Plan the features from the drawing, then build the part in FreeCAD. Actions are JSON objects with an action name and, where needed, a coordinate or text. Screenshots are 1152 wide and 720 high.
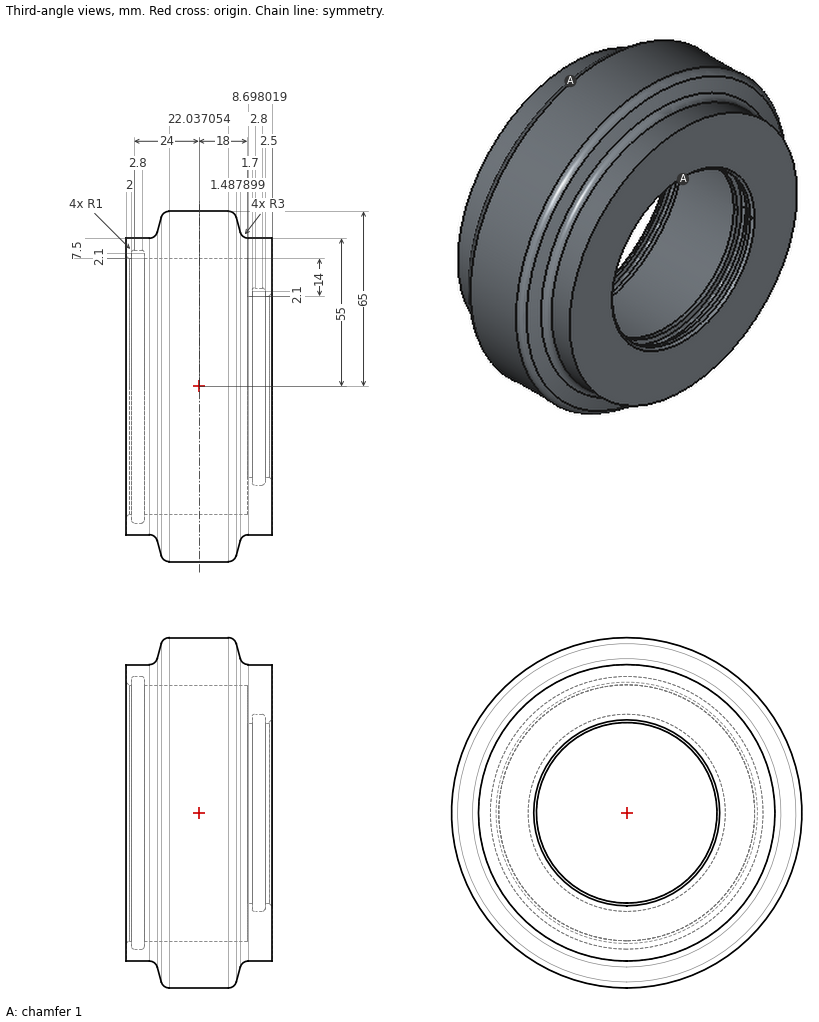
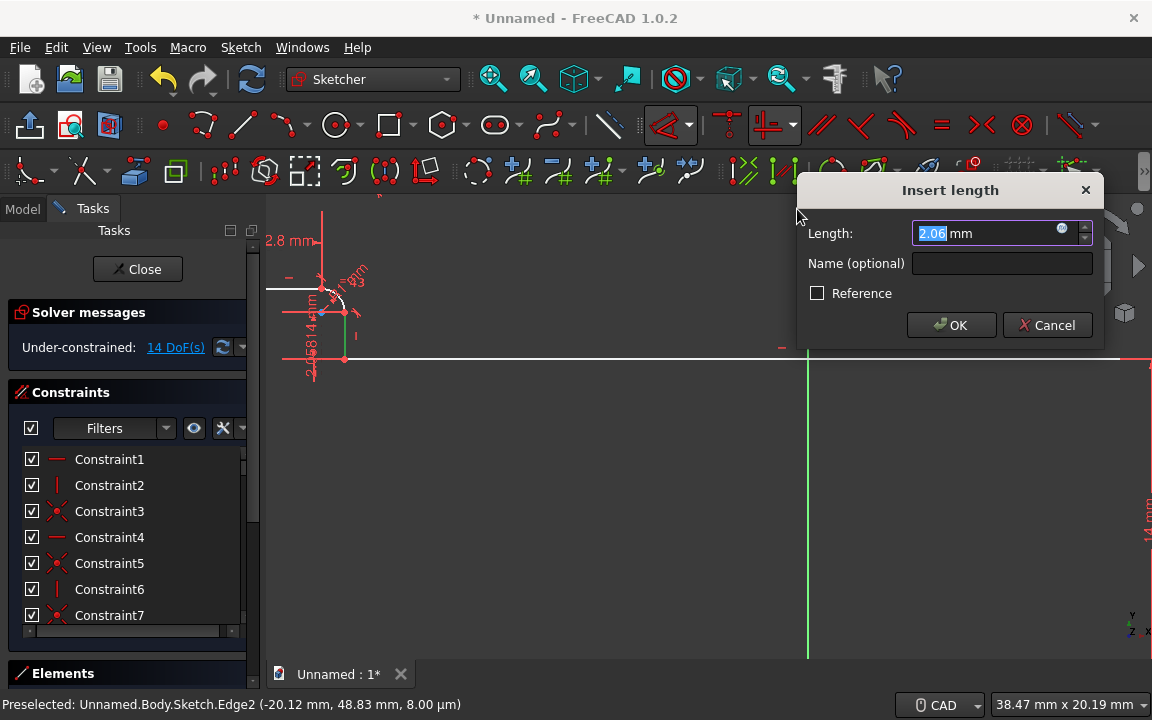
{"action": "type", "text": "2.1"}
{"action": "key", "text": "Return"}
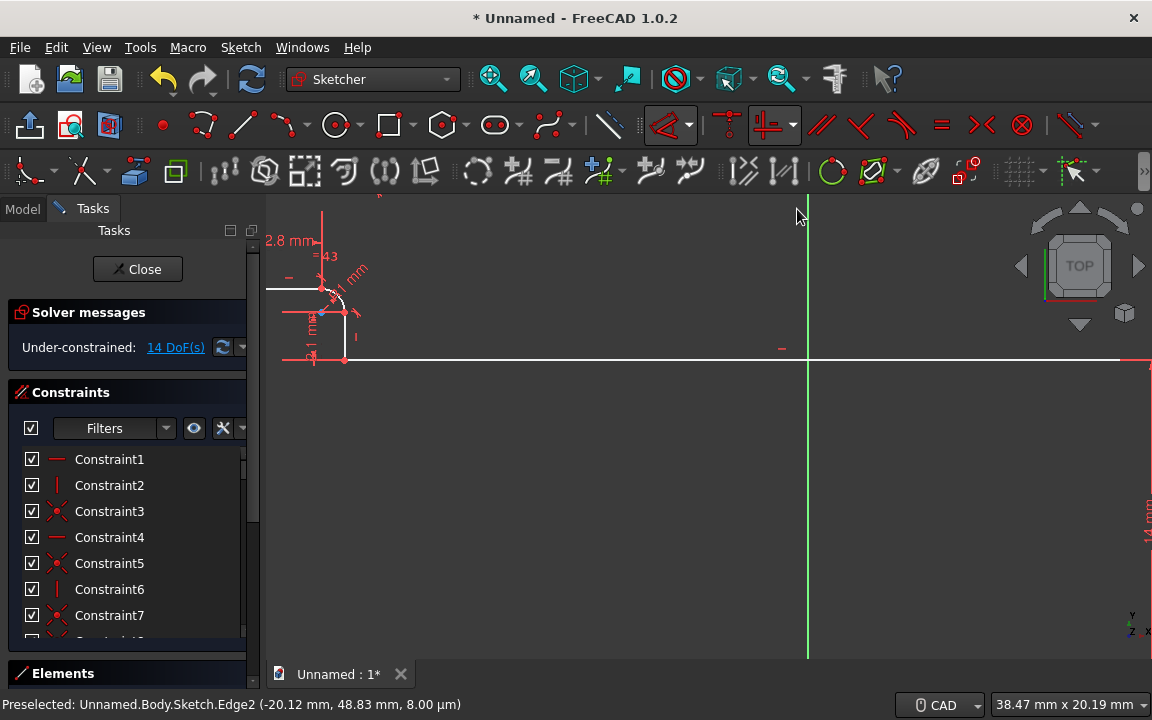
{"action": "scroll", "coordinate": [598, 357], "scroll_direction": "down", "scroll_amount": 8}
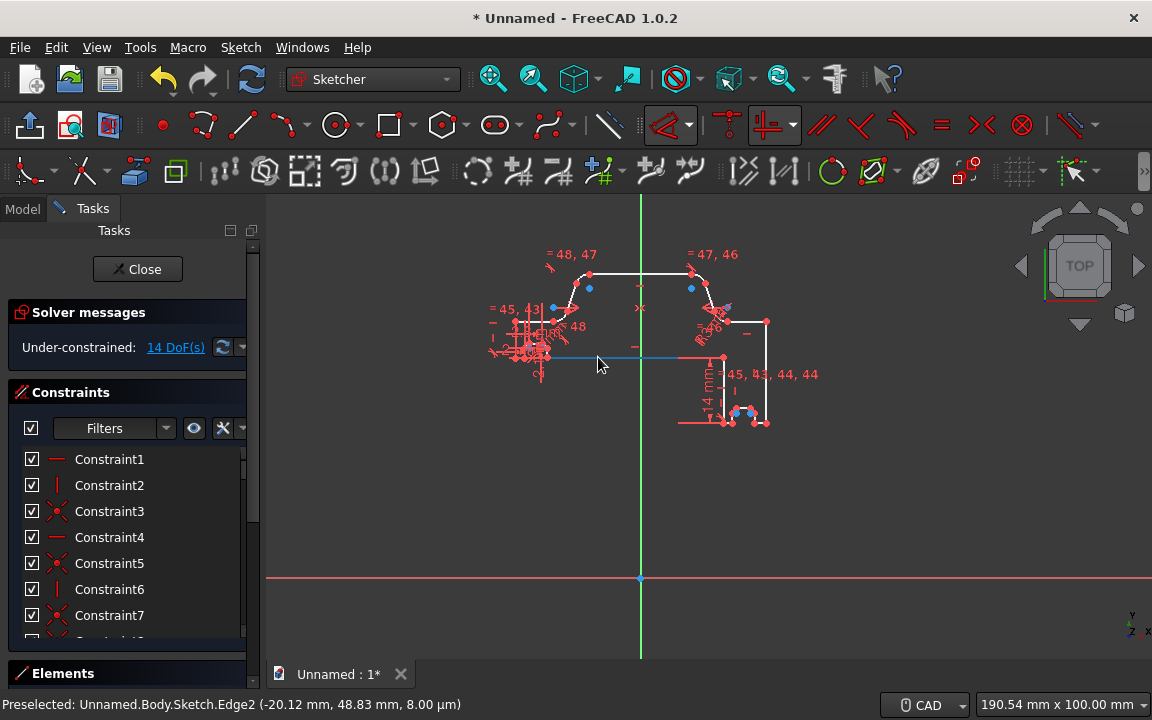
{"action": "scroll", "coordinate": [726, 423], "scroll_direction": "up", "scroll_amount": 9}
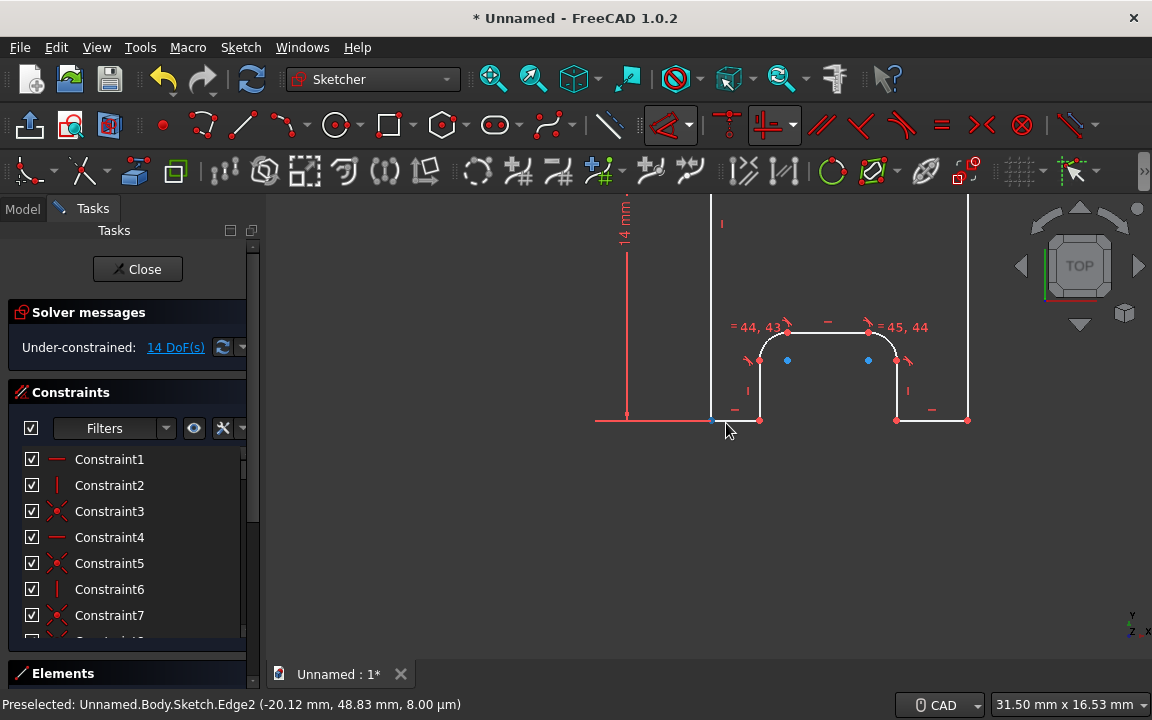
{"action": "left_click", "coordinate": [726, 421]}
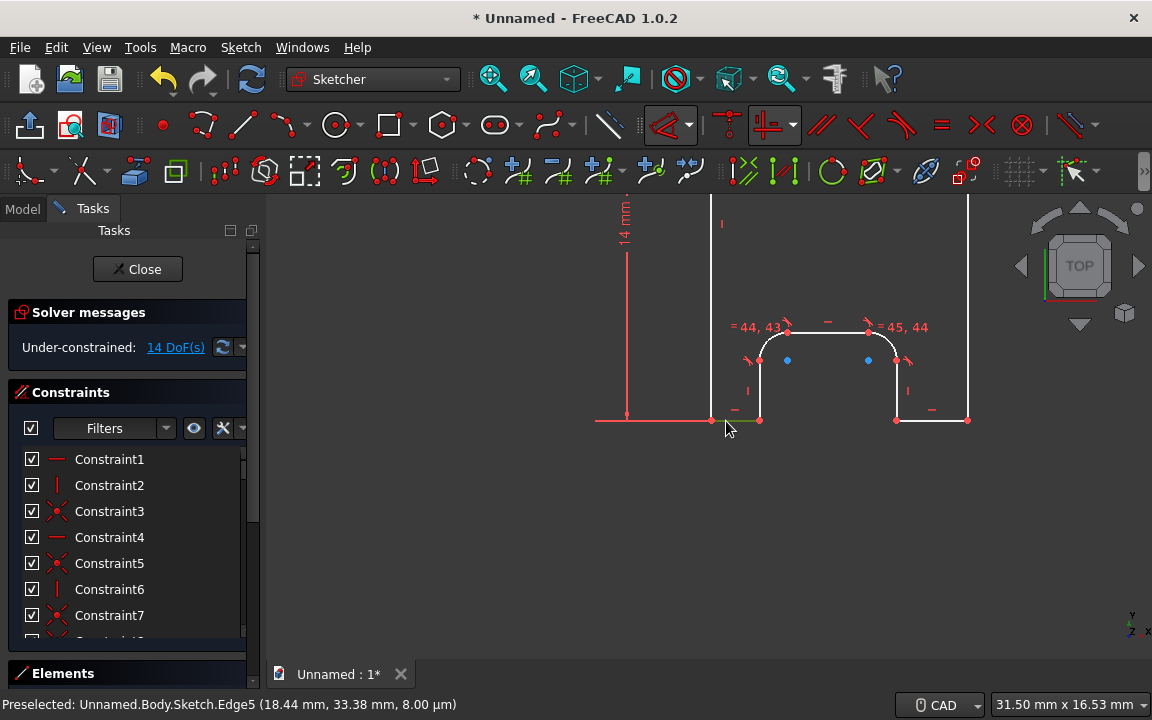
{"action": "key", "text": "l"}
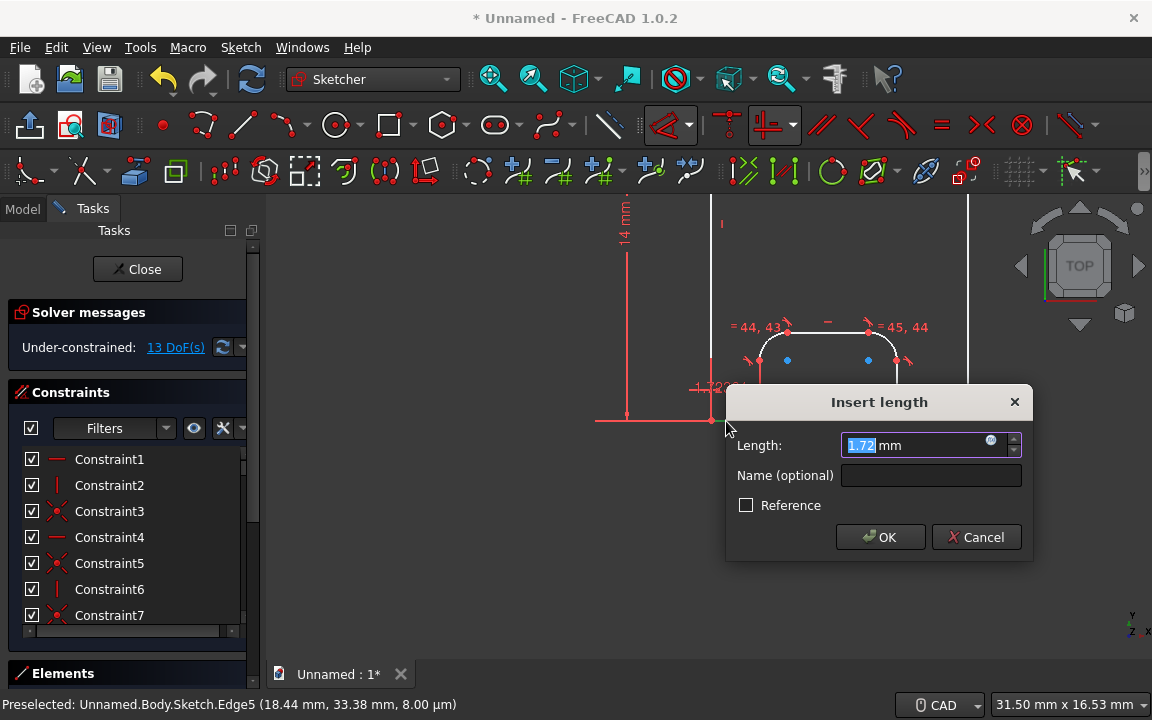
{"action": "type", "text": "1.7"}
{"action": "key", "text": "Return"}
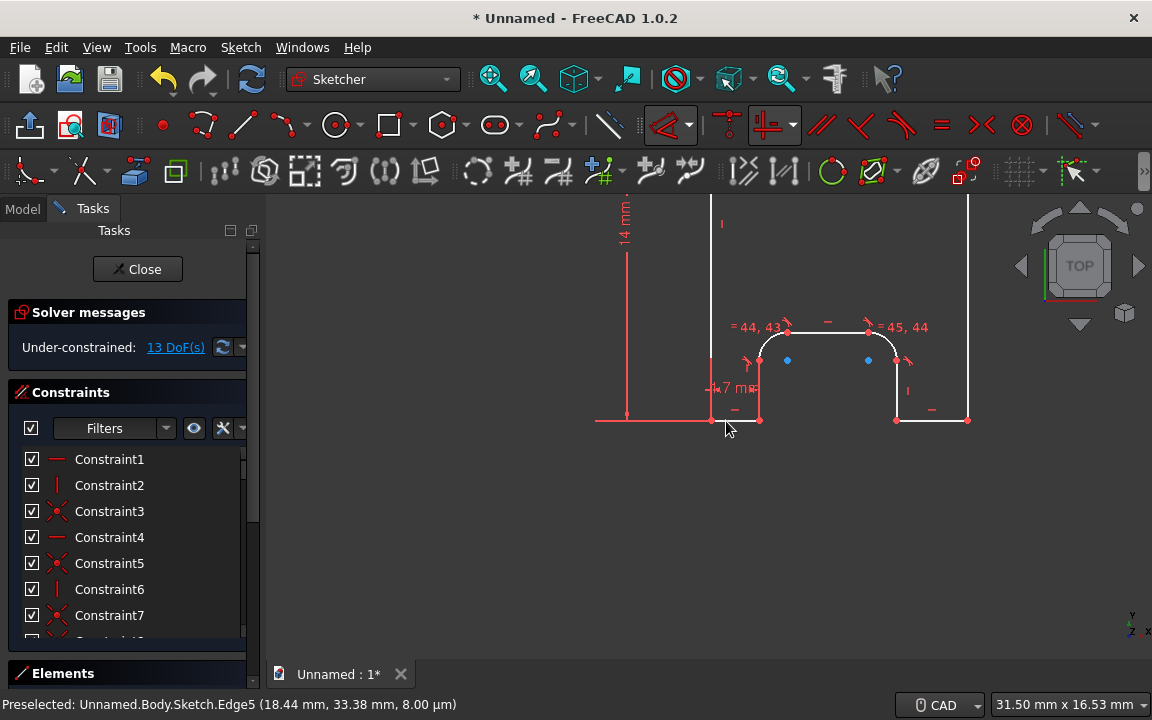
{"action": "left_click", "coordinate": [759, 403]}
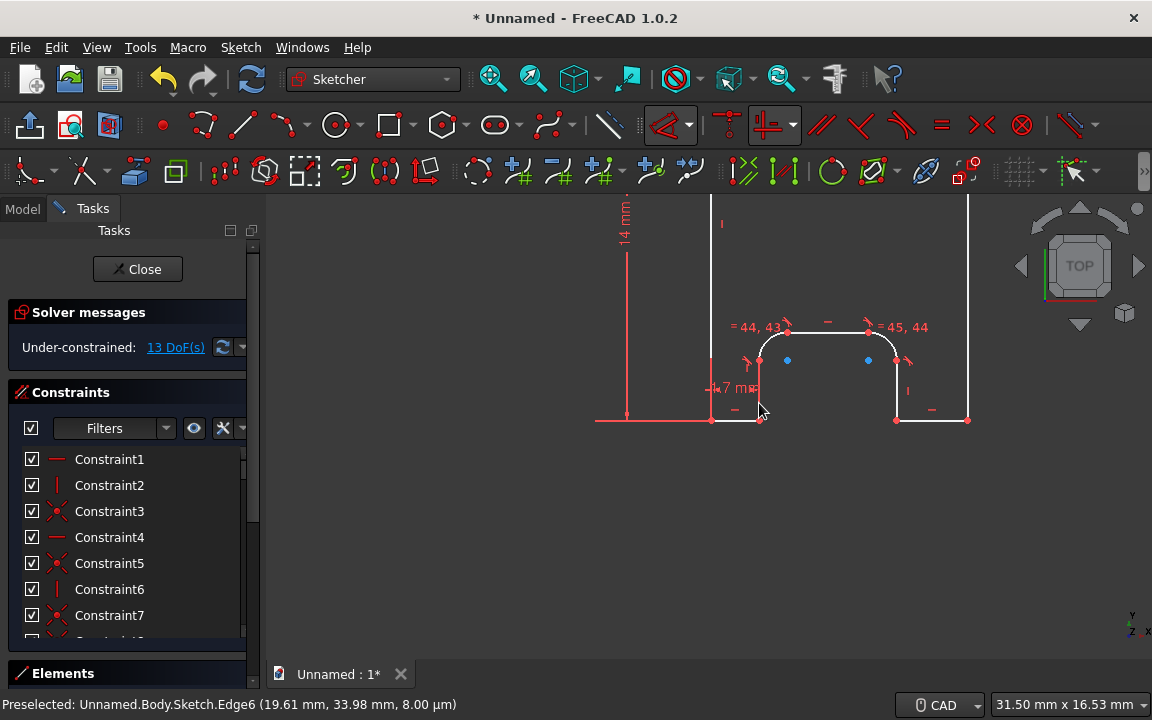
{"action": "key", "text": "i"}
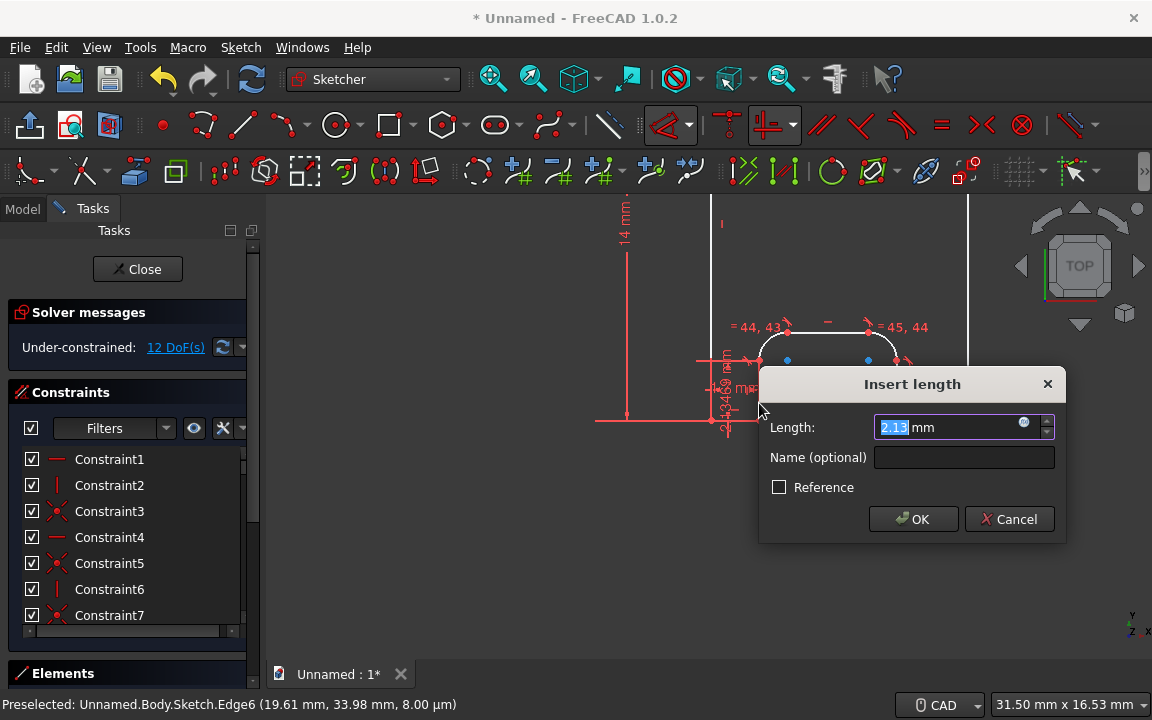
{"action": "type", "text": "2.1"}
{"action": "key", "text": "Return"}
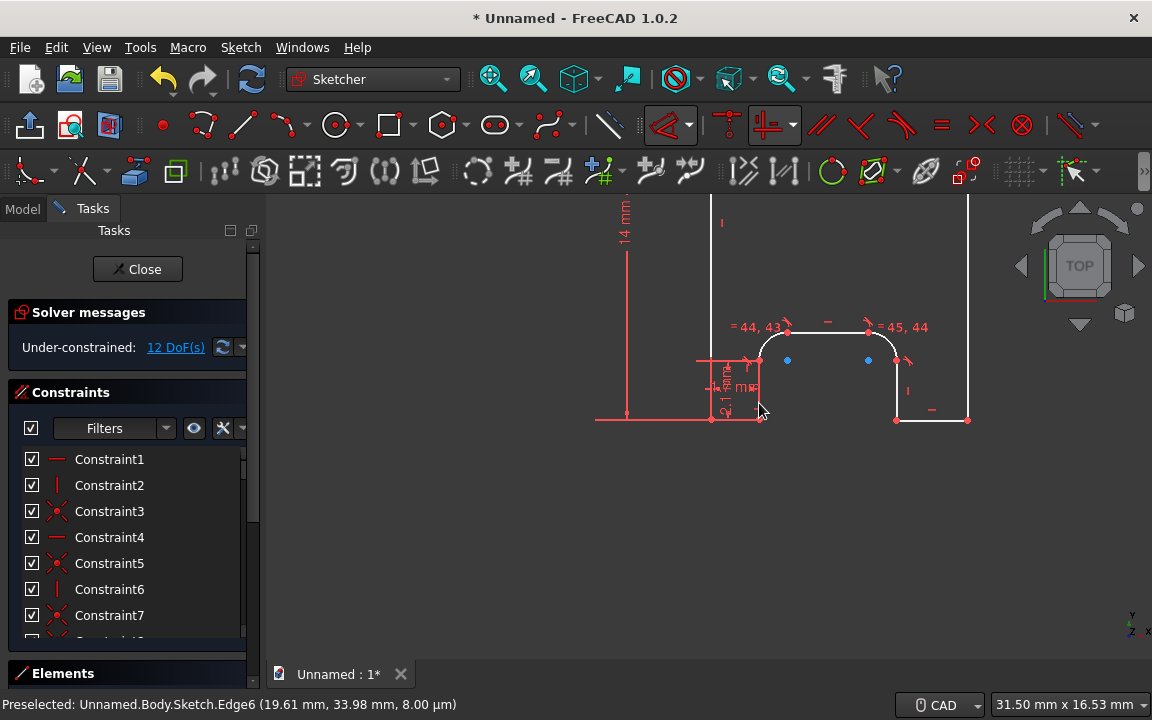
{"action": "left_click", "coordinate": [812, 333]}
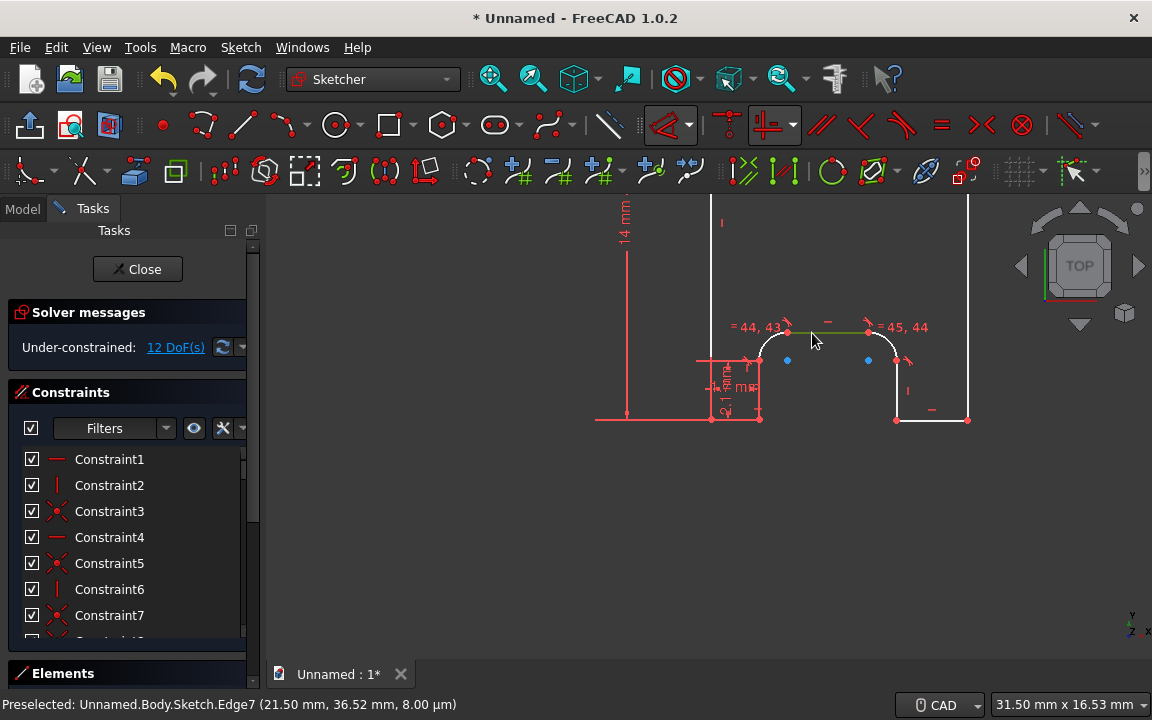
{"action": "key", "text": "l"}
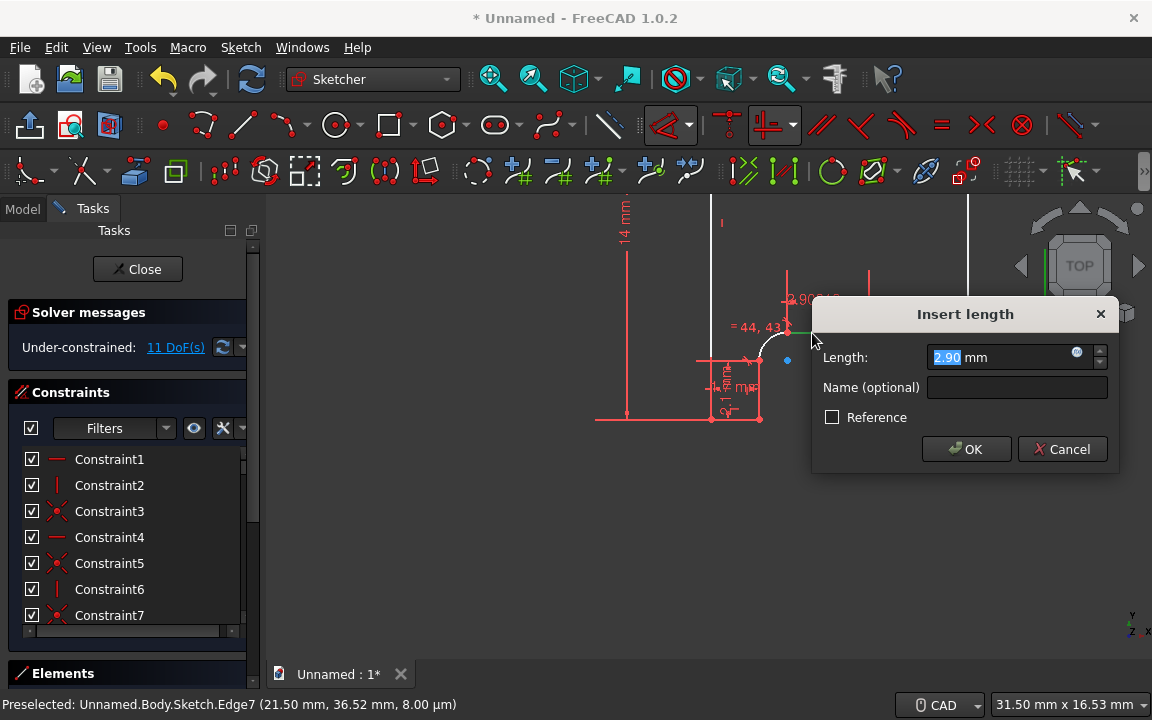
{"action": "type", "text": "2.8"}
{"action": "key", "text": "Return"}